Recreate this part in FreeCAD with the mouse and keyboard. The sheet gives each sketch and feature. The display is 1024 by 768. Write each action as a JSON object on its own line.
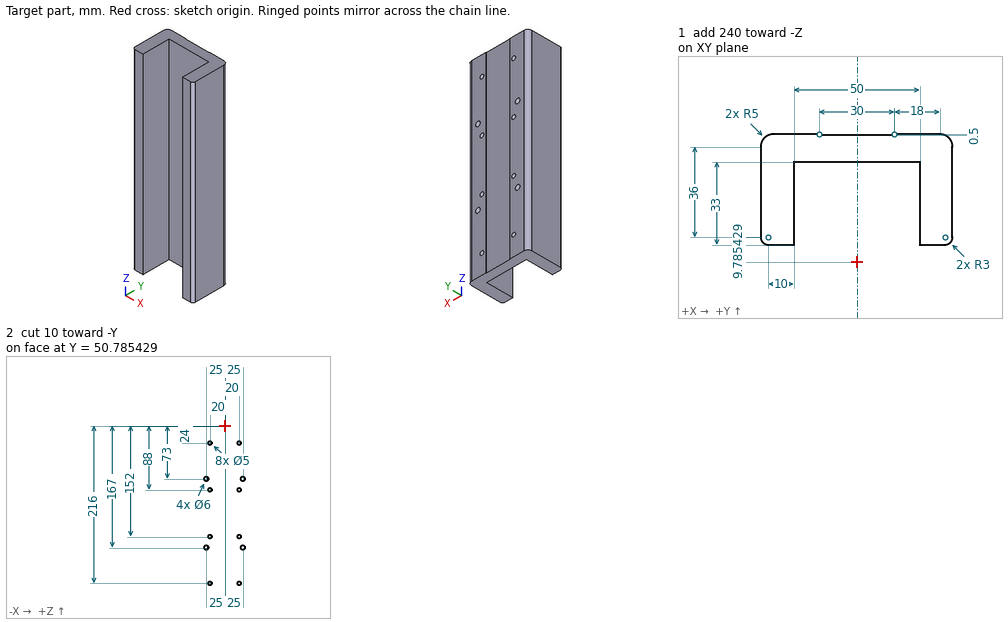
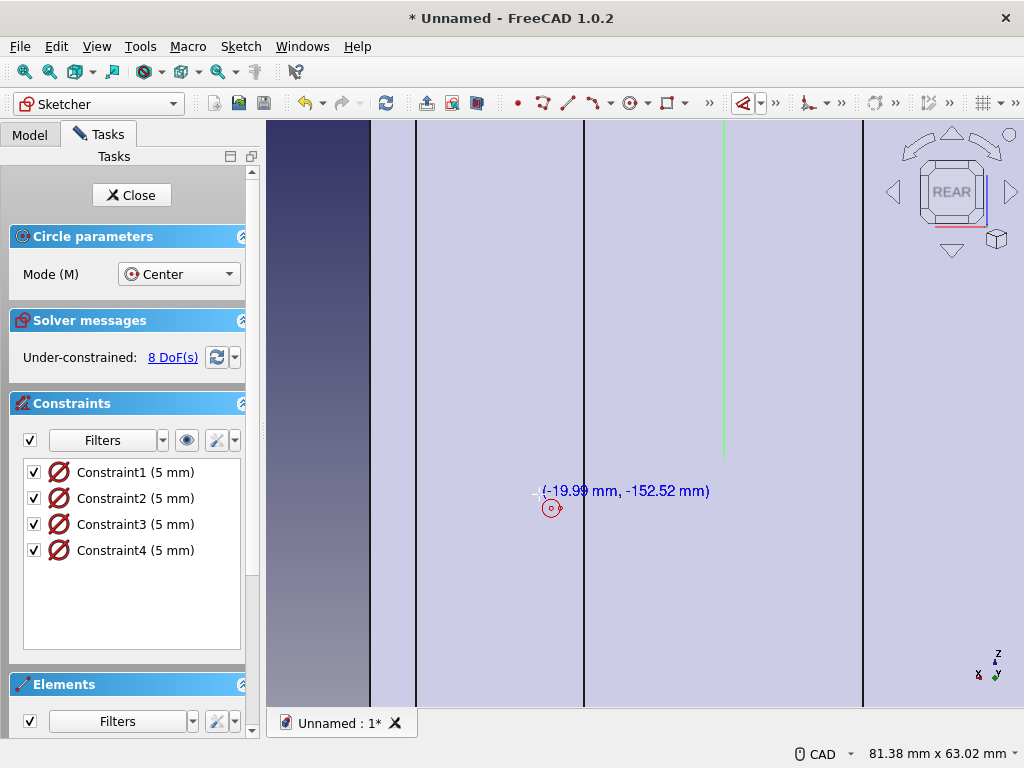
{"action": "scroll", "coordinate": [539, 494], "scroll_direction": "down", "scroll_amount": 8}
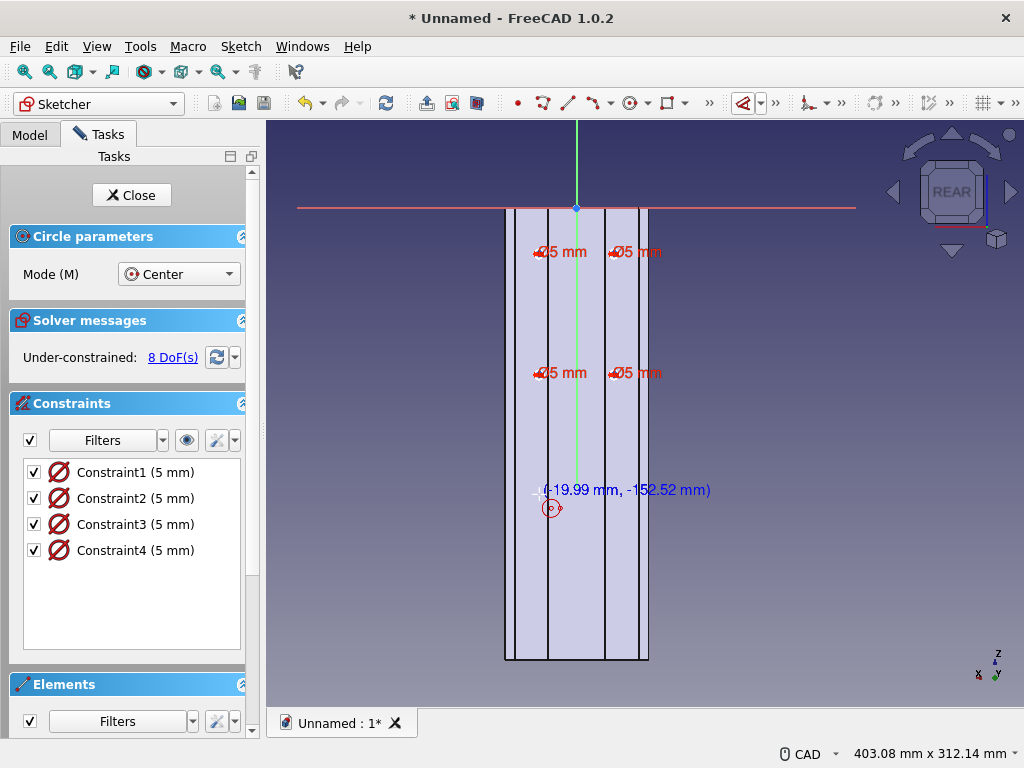
{"action": "left_click", "coordinate": [539, 494]}
{"action": "mouse_move", "coordinate": [542, 491]}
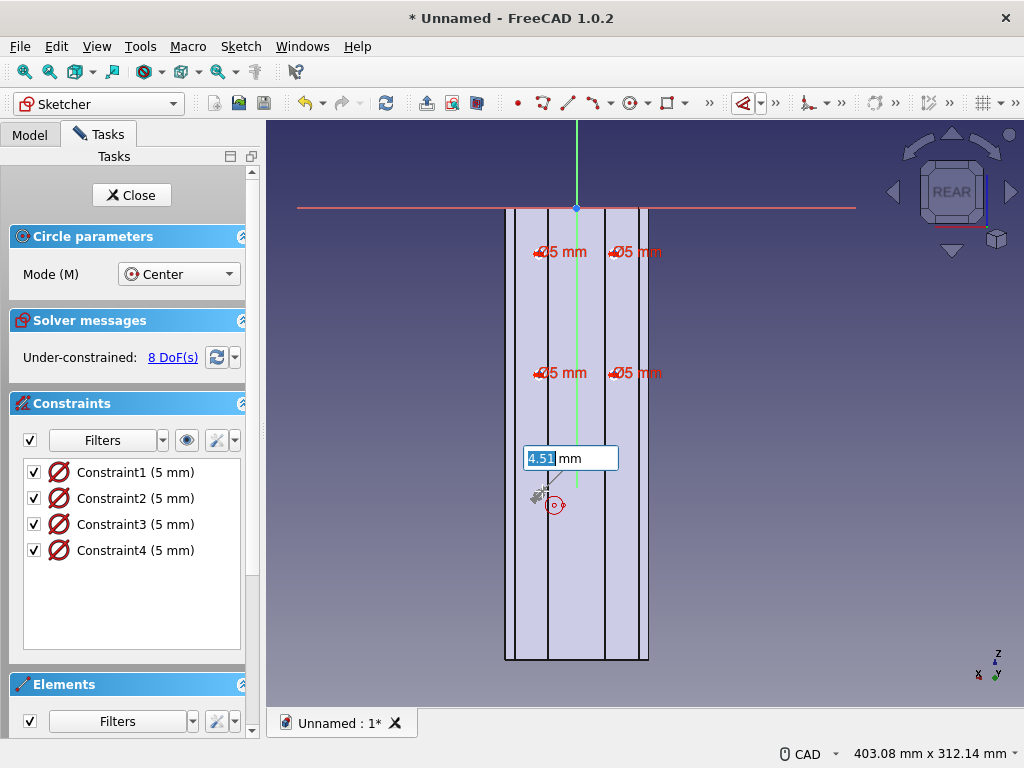
{"action": "type", "text": "5"}
{"action": "key", "text": "Return"}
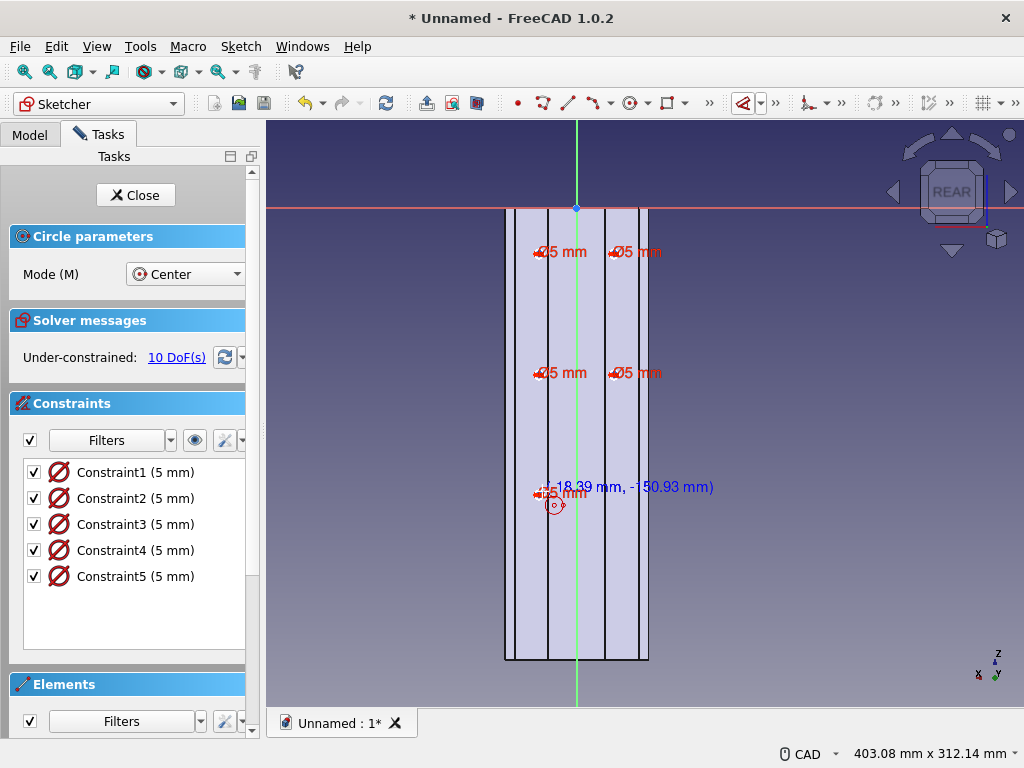
{"action": "scroll", "coordinate": [614, 494], "scroll_direction": "up", "scroll_amount": 8}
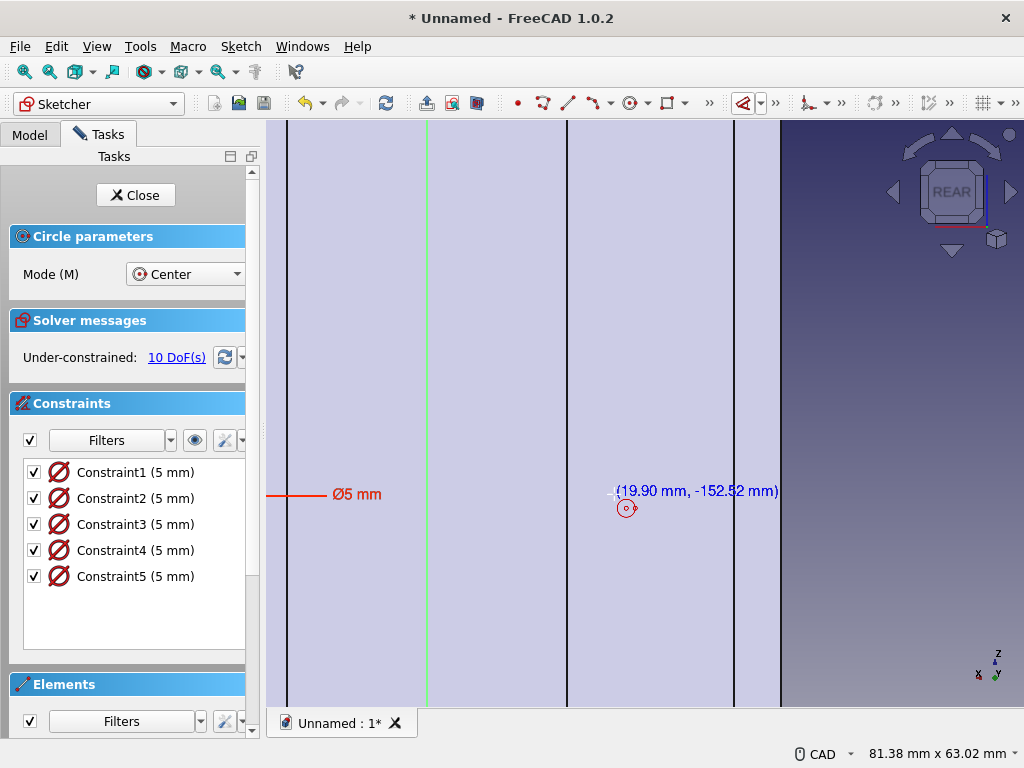
{"action": "scroll", "coordinate": [614, 494], "scroll_direction": "down", "scroll_amount": 8}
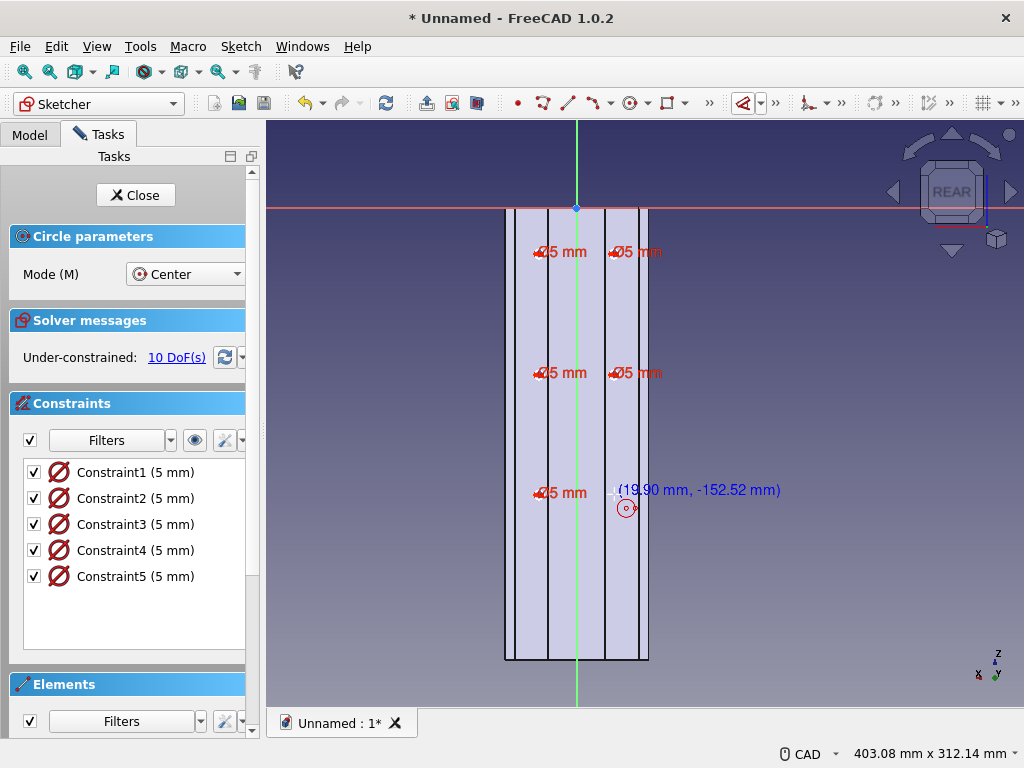
{"action": "left_click", "coordinate": [614, 494]}
{"action": "mouse_move", "coordinate": [618, 491]}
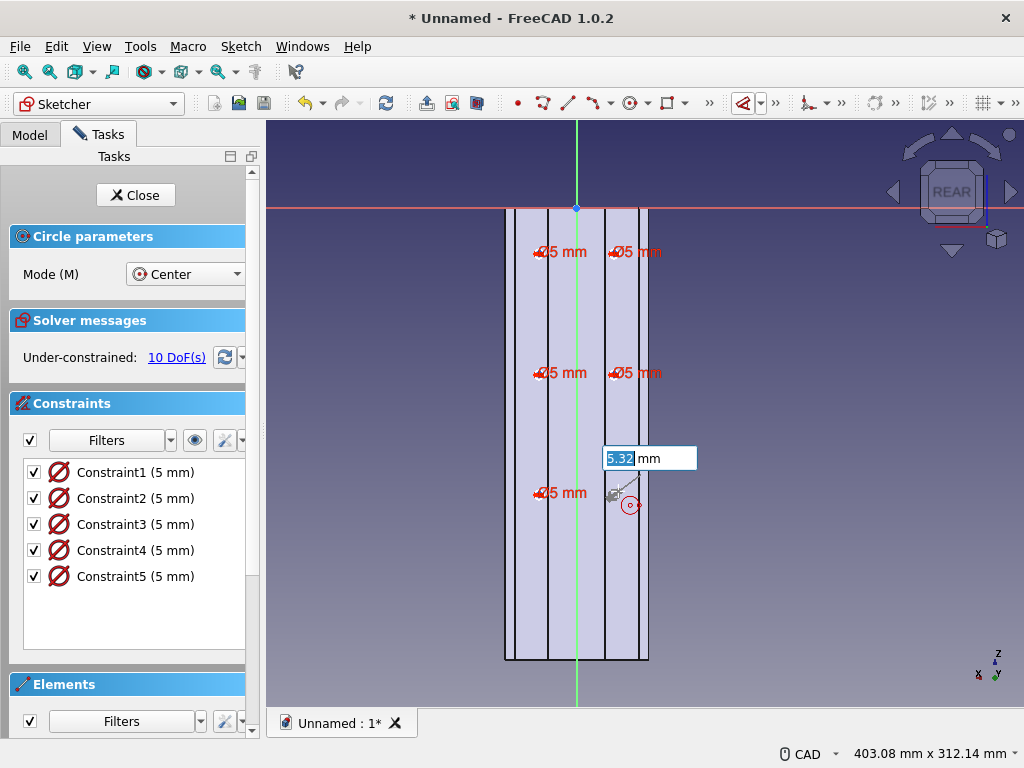
{"action": "type", "text": "5"}
{"action": "key", "text": "Return"}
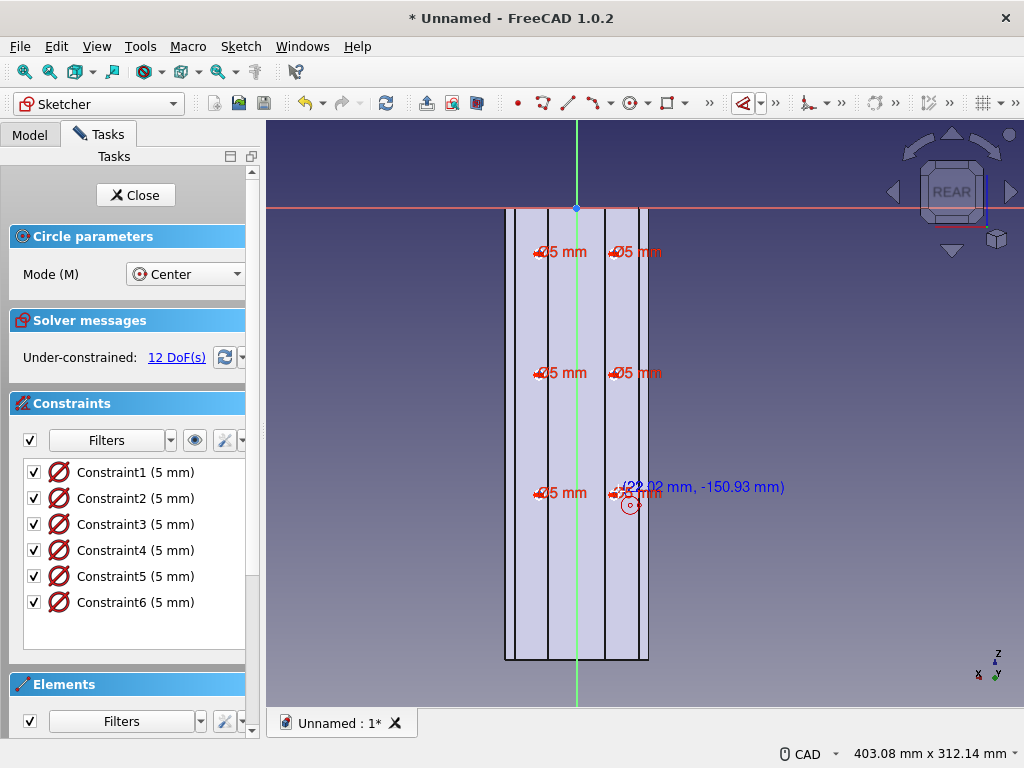
{"action": "scroll", "coordinate": [539, 614], "scroll_direction": "up", "scroll_amount": 8}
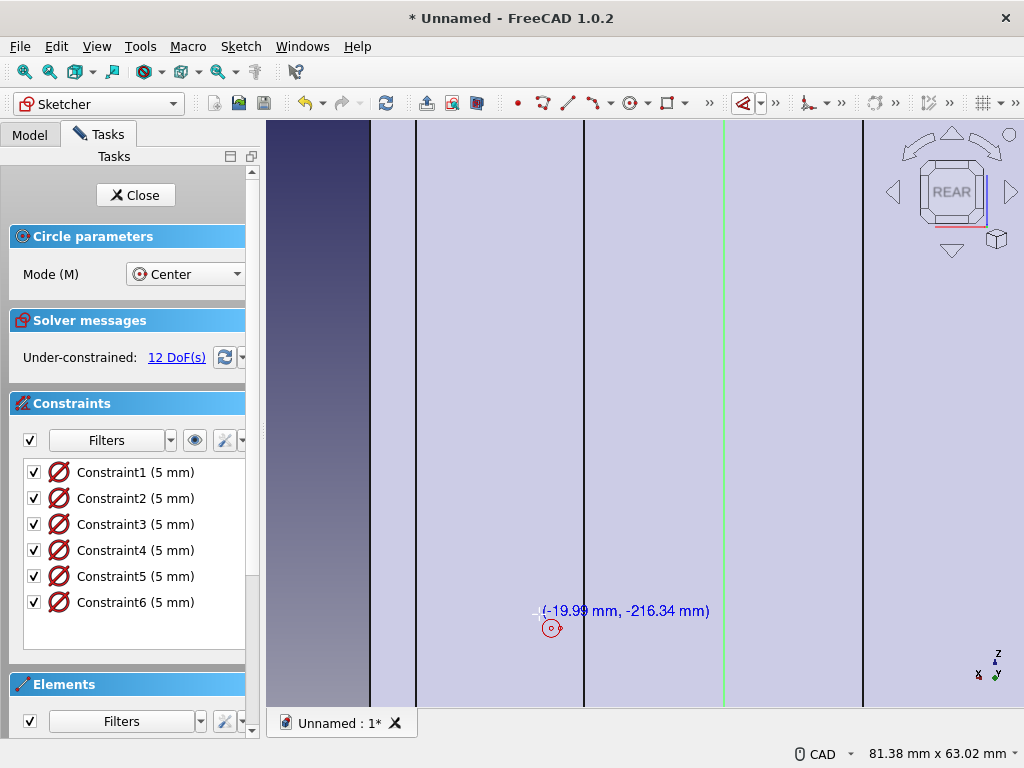
{"action": "scroll", "coordinate": [539, 615], "scroll_direction": "down", "scroll_amount": 8}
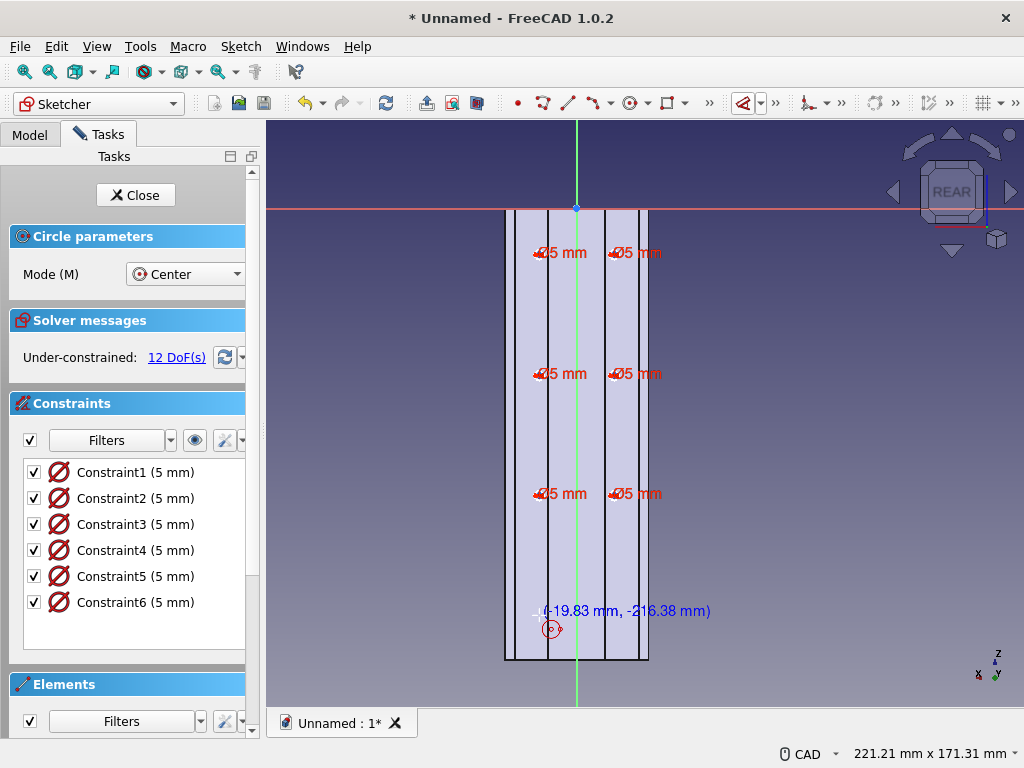
{"action": "left_click", "coordinate": [539, 615]}
{"action": "mouse_move", "coordinate": [542, 612]}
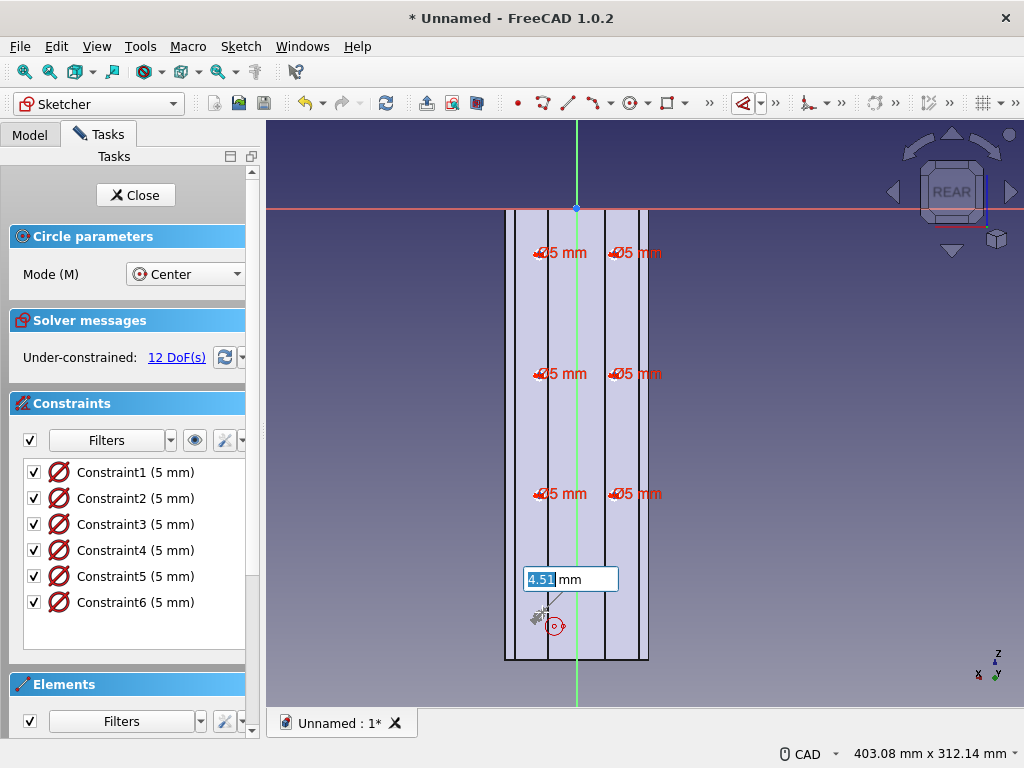
{"action": "type", "text": "5"}
{"action": "key", "text": "Return"}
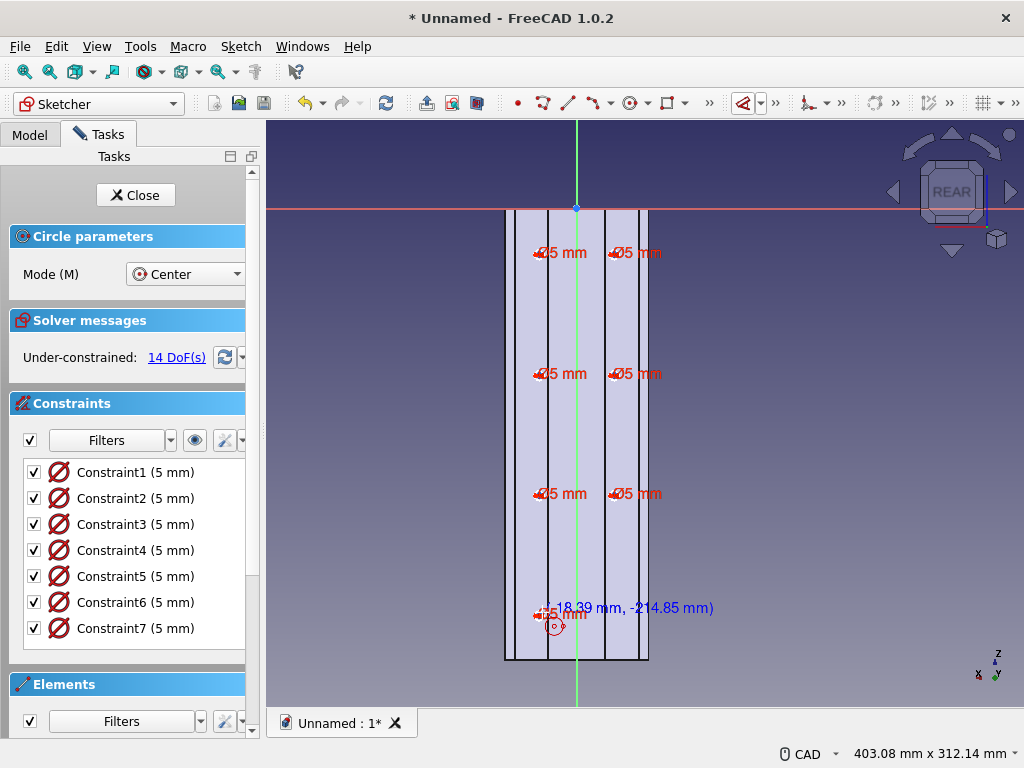
{"action": "scroll", "coordinate": [614, 615], "scroll_direction": "up", "scroll_amount": 8}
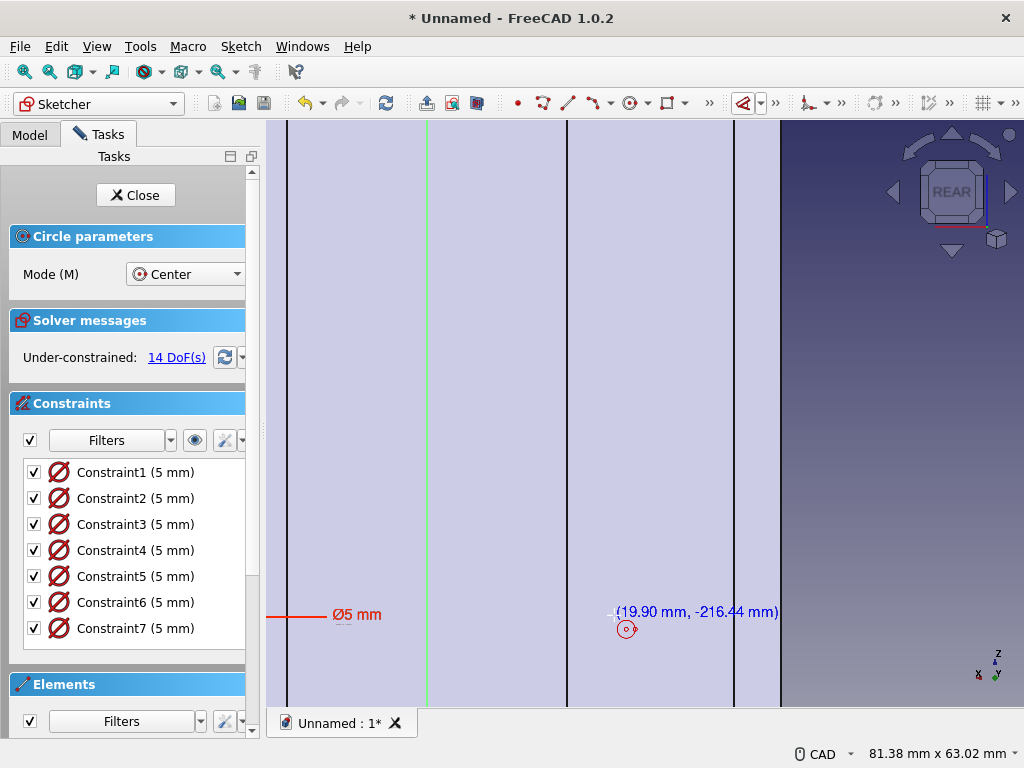
{"action": "scroll", "coordinate": [614, 615], "scroll_direction": "down", "scroll_amount": 8}